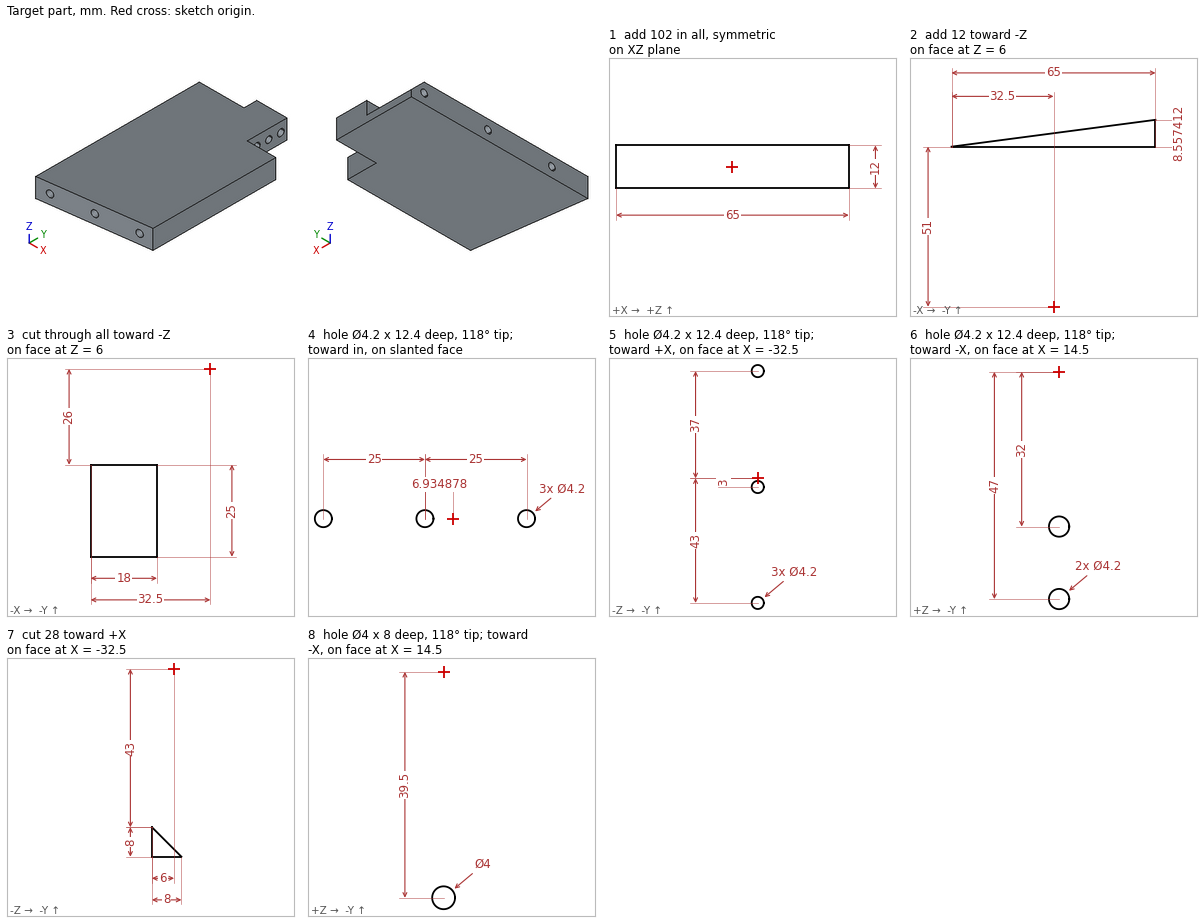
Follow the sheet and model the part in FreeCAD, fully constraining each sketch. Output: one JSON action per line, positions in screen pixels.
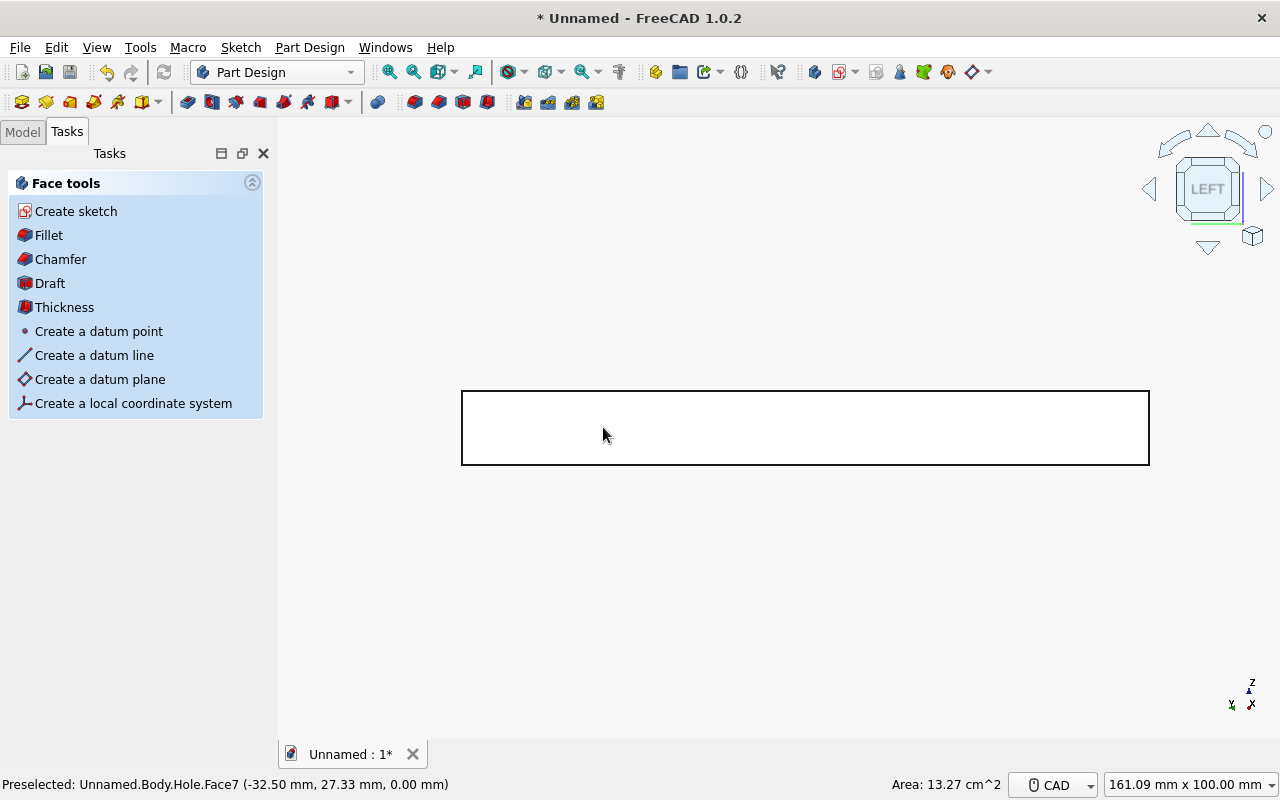
{"action": "left_click", "coordinate": [840, 72]}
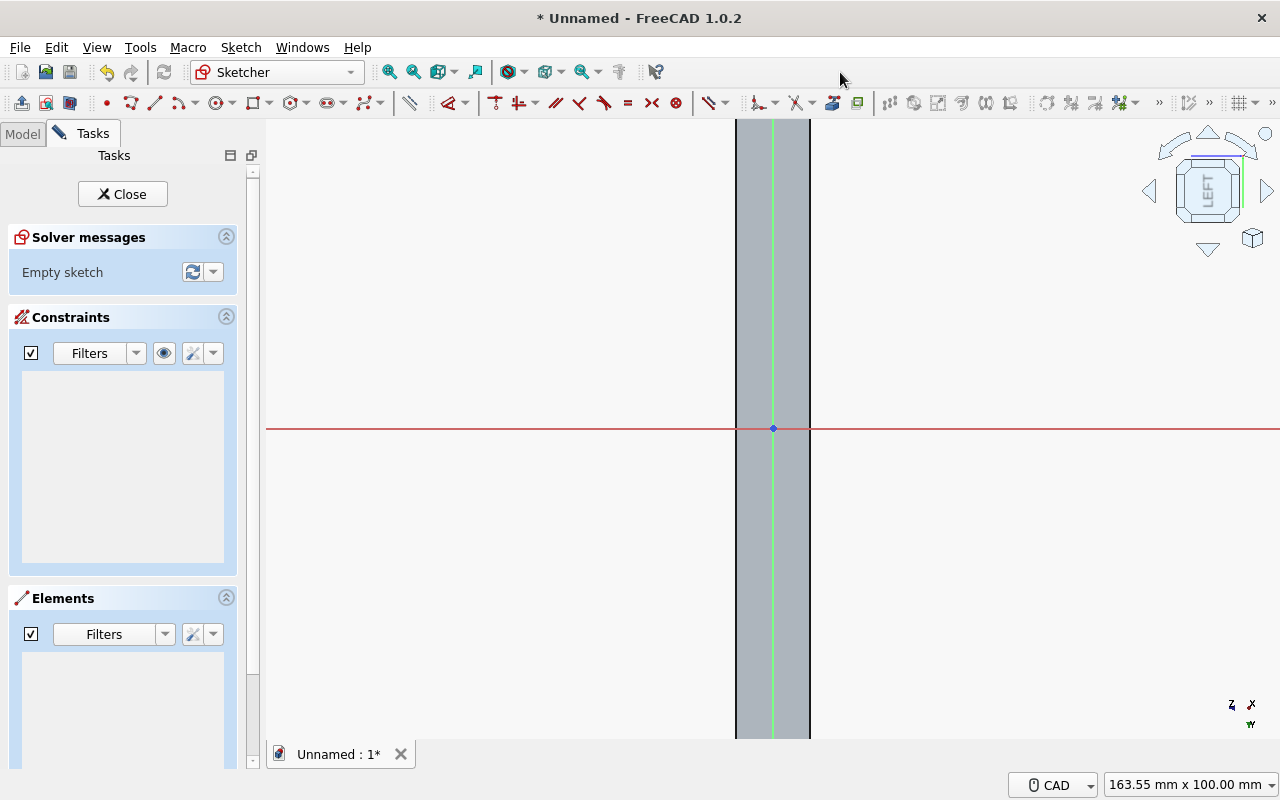
{"action": "scroll", "coordinate": [395, 345], "scroll_direction": "down", "scroll_amount": 1}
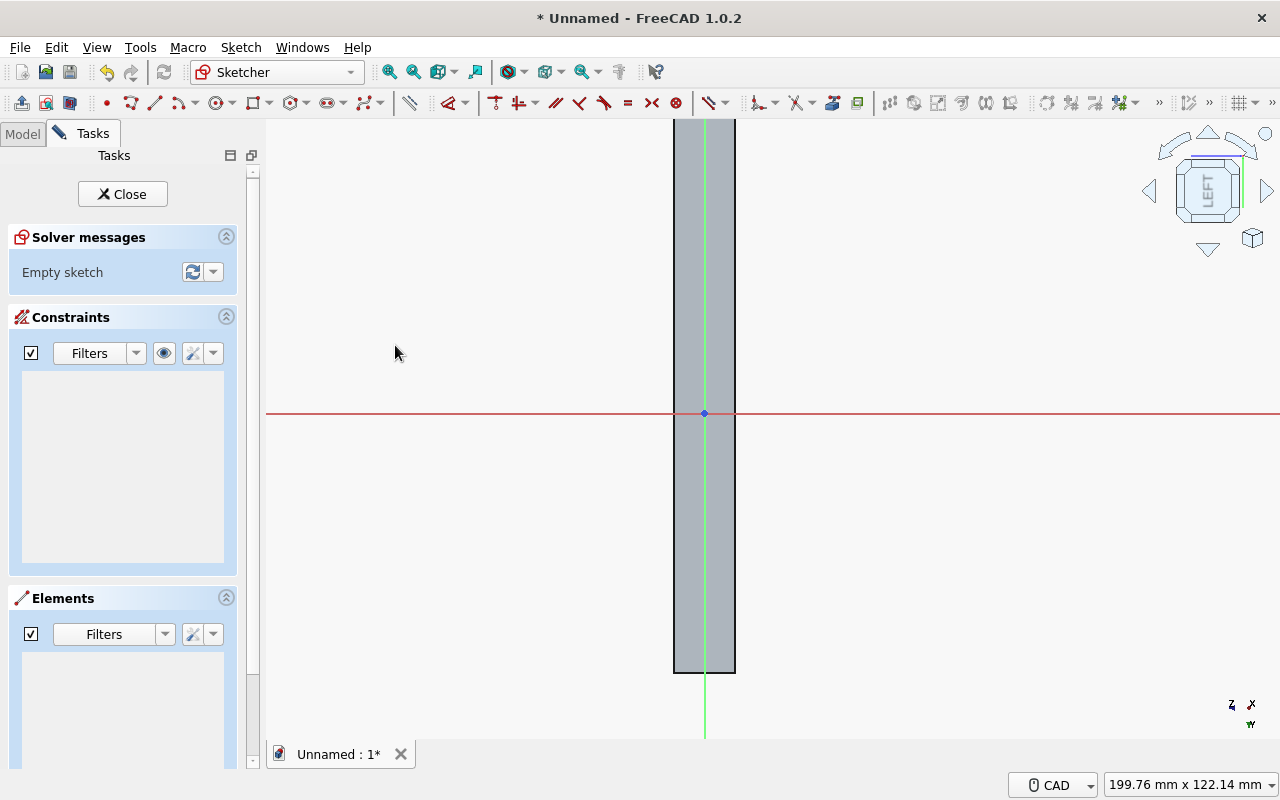
{"action": "key", "text": "g c"}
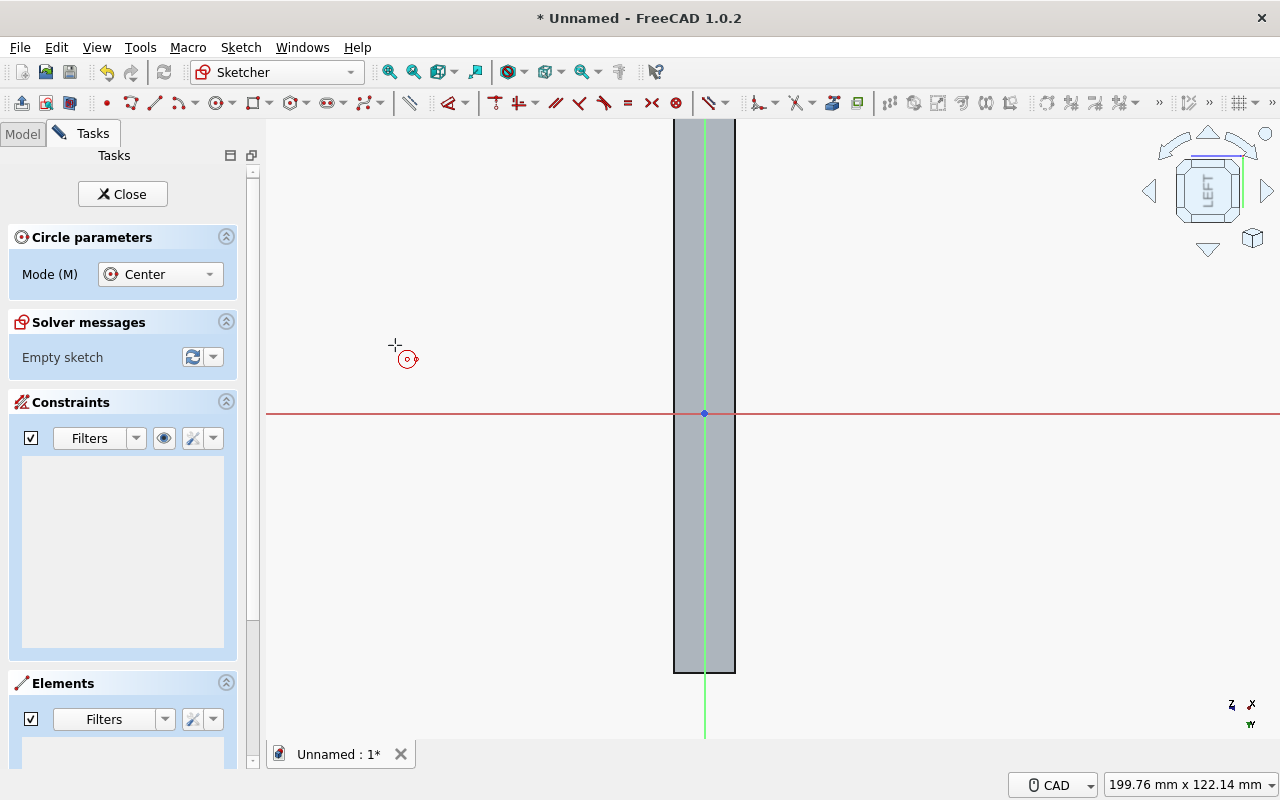
{"action": "scroll", "coordinate": [705, 632], "scroll_direction": "up", "scroll_amount": 4}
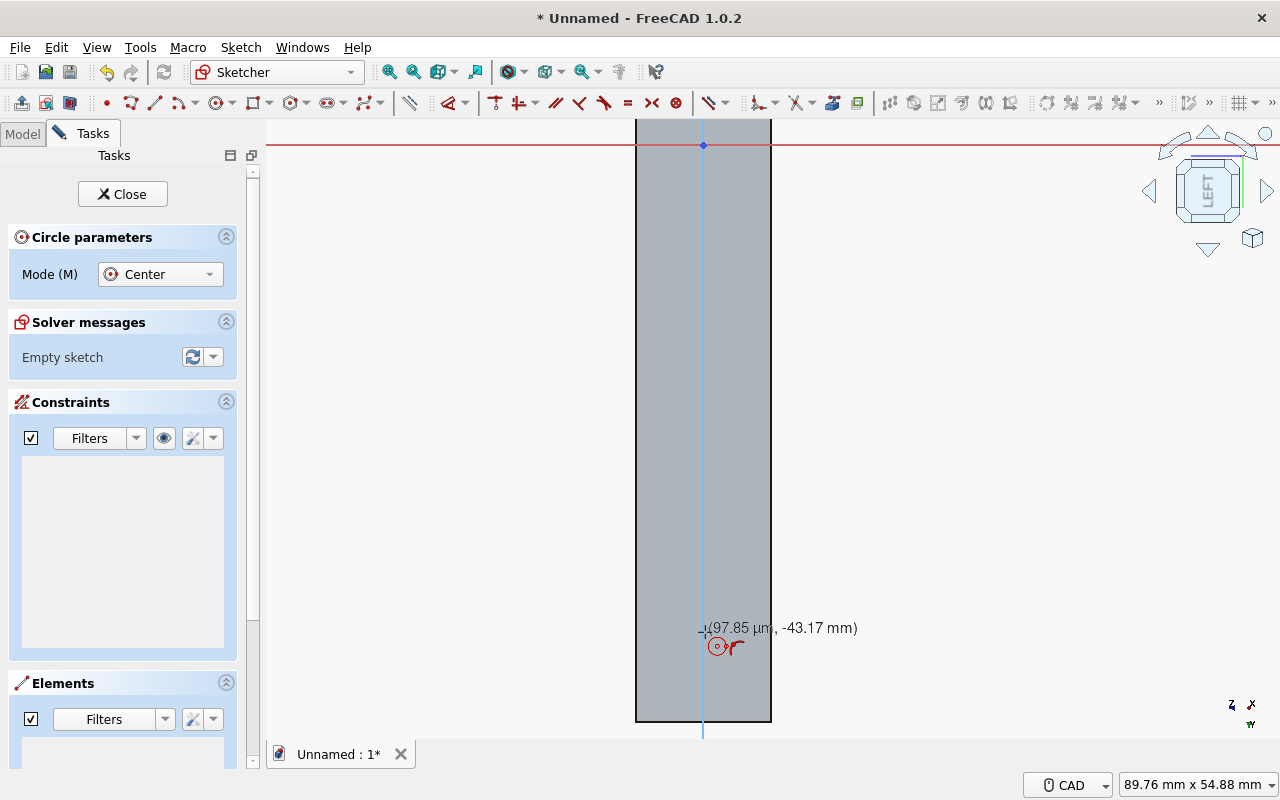
{"action": "left_click", "coordinate": [703, 631]}
{"action": "mouse_move", "coordinate": [720, 614]}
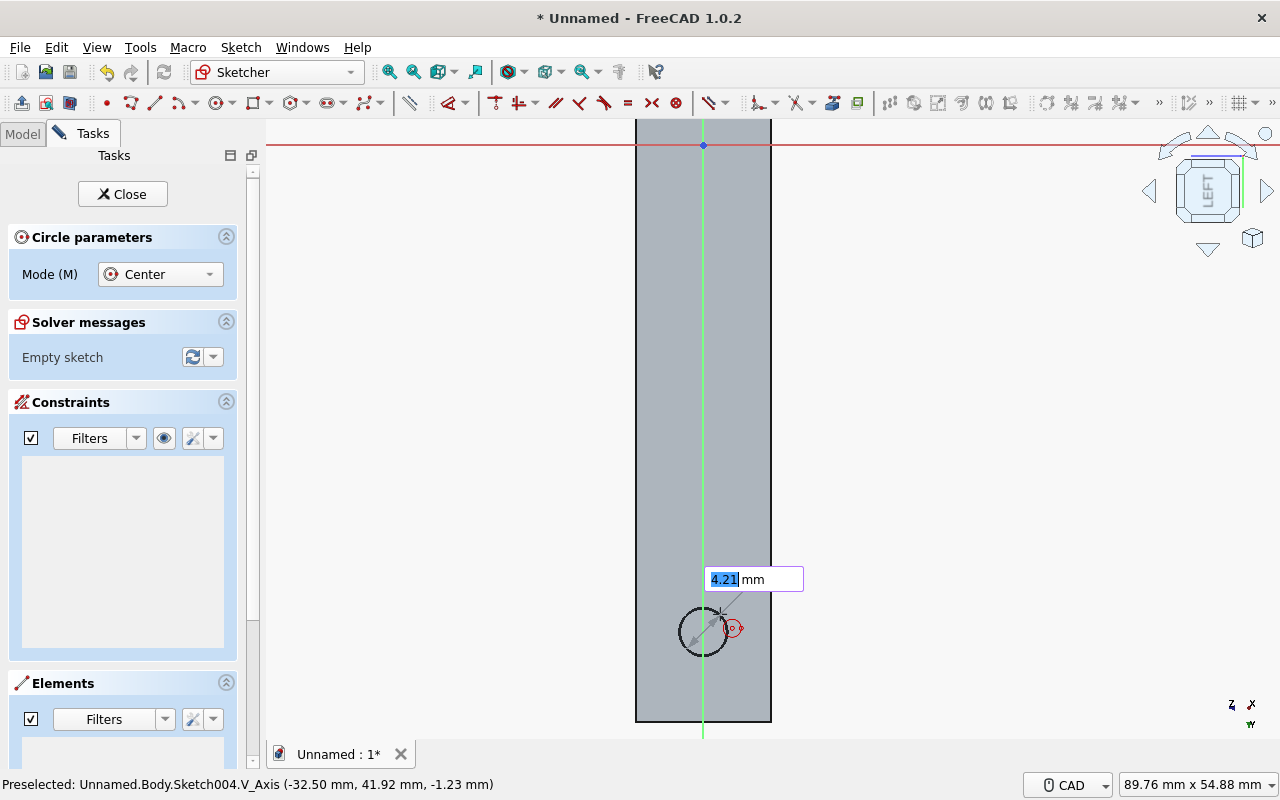
{"action": "type", "text": "4.2"}
{"action": "key", "text": "Return"}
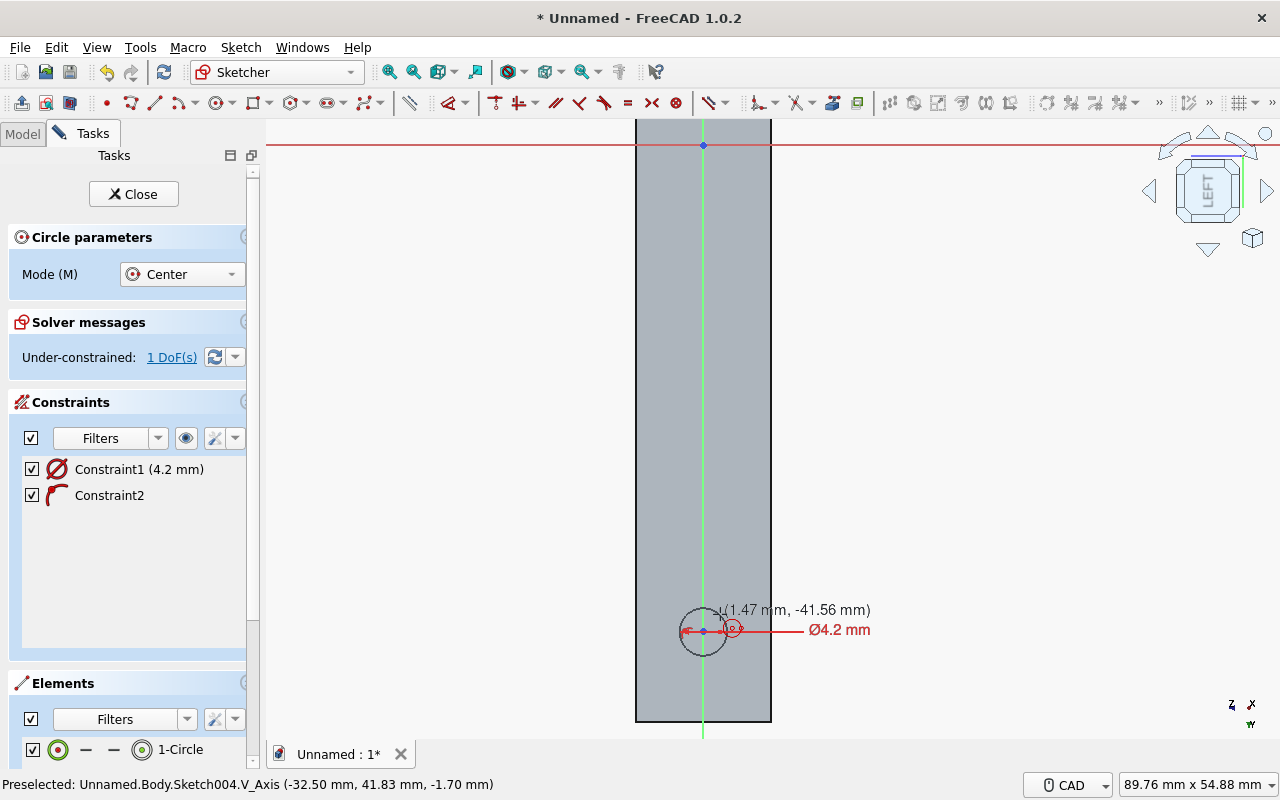
{"action": "left_click", "coordinate": [703, 179]}
{"action": "mouse_move", "coordinate": [720, 163]}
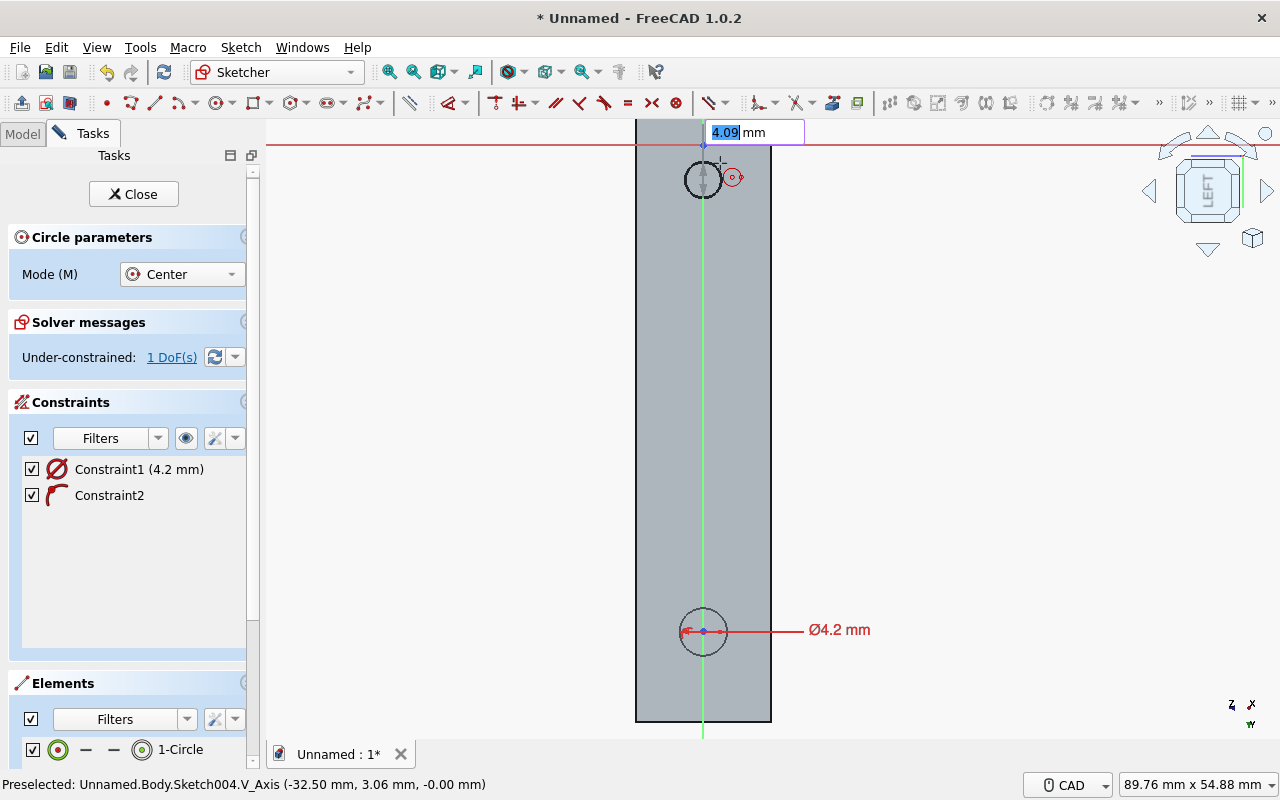
{"action": "type", "text": "4.2"}
{"action": "key", "text": "Return"}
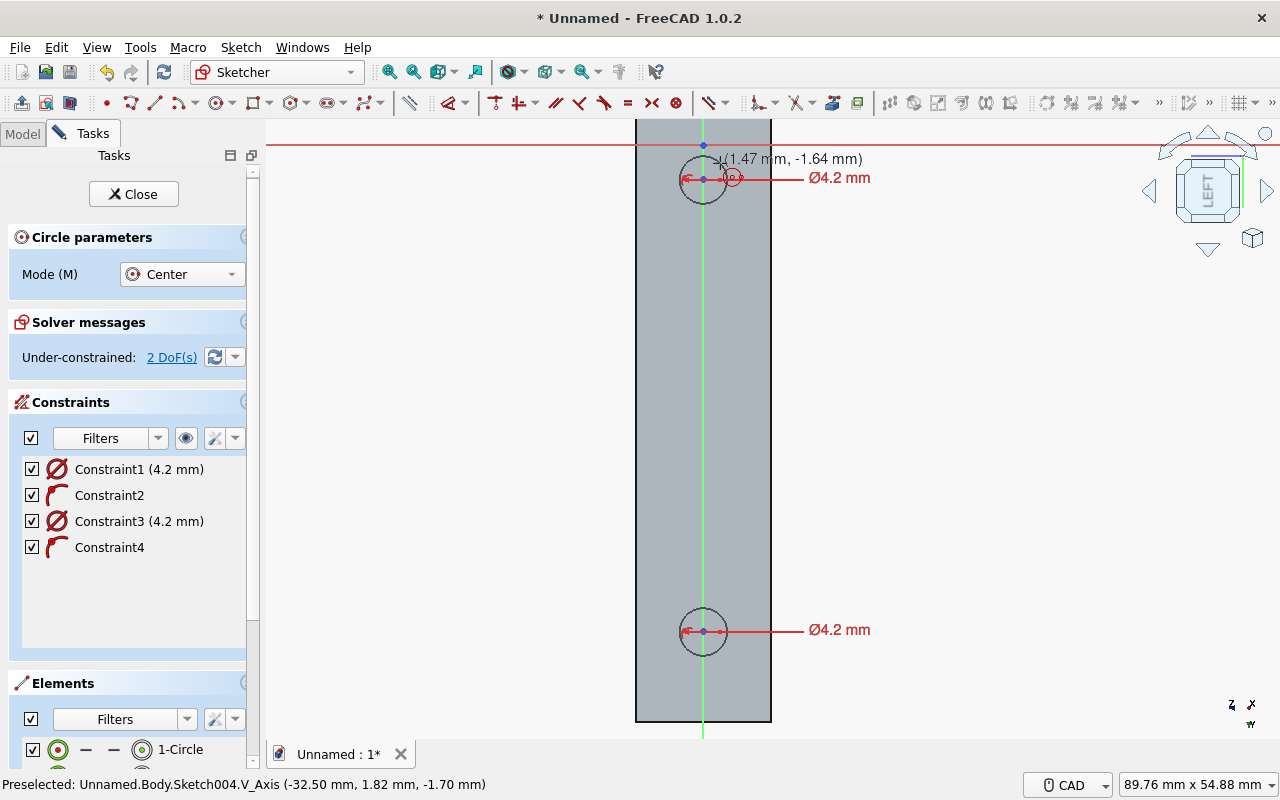
{"action": "scroll", "coordinate": [705, 633], "scroll_direction": "down", "scroll_amount": 4}